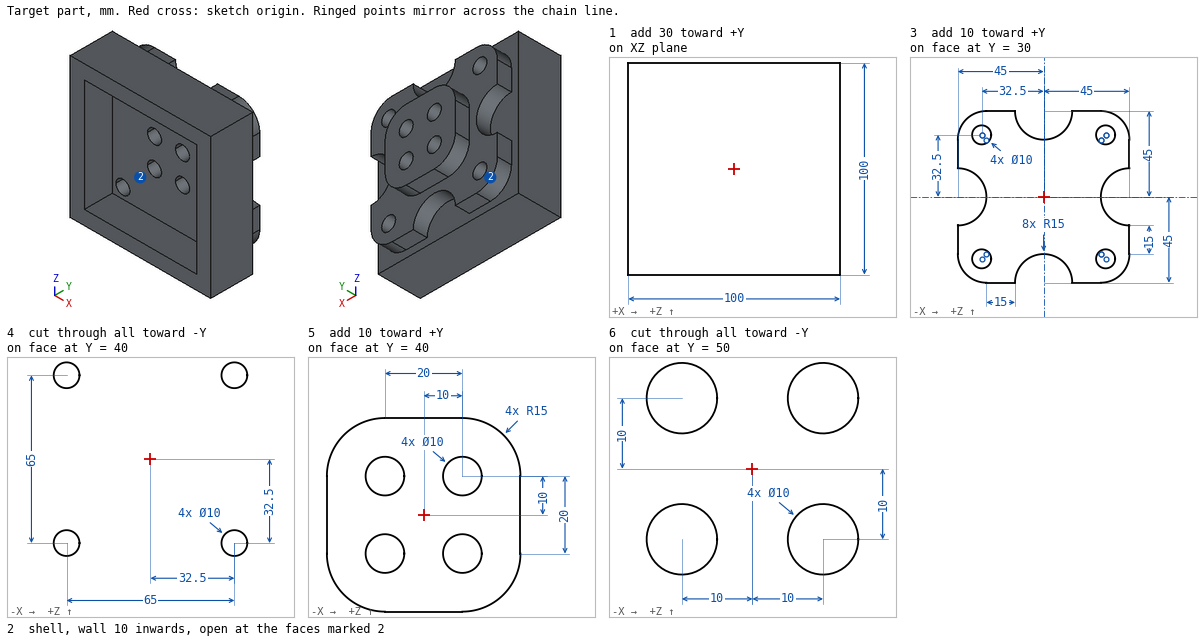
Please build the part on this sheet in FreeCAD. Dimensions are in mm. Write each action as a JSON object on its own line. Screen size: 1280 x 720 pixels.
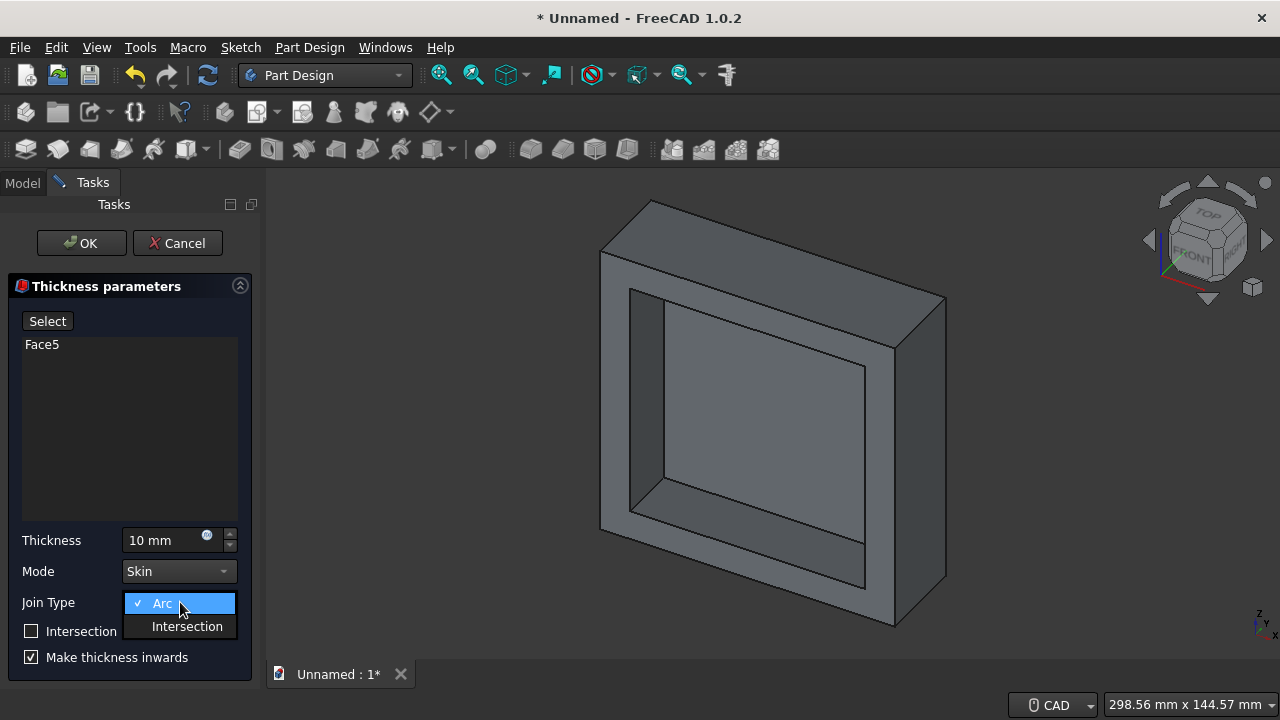
{"action": "left_click", "coordinate": [179, 626]}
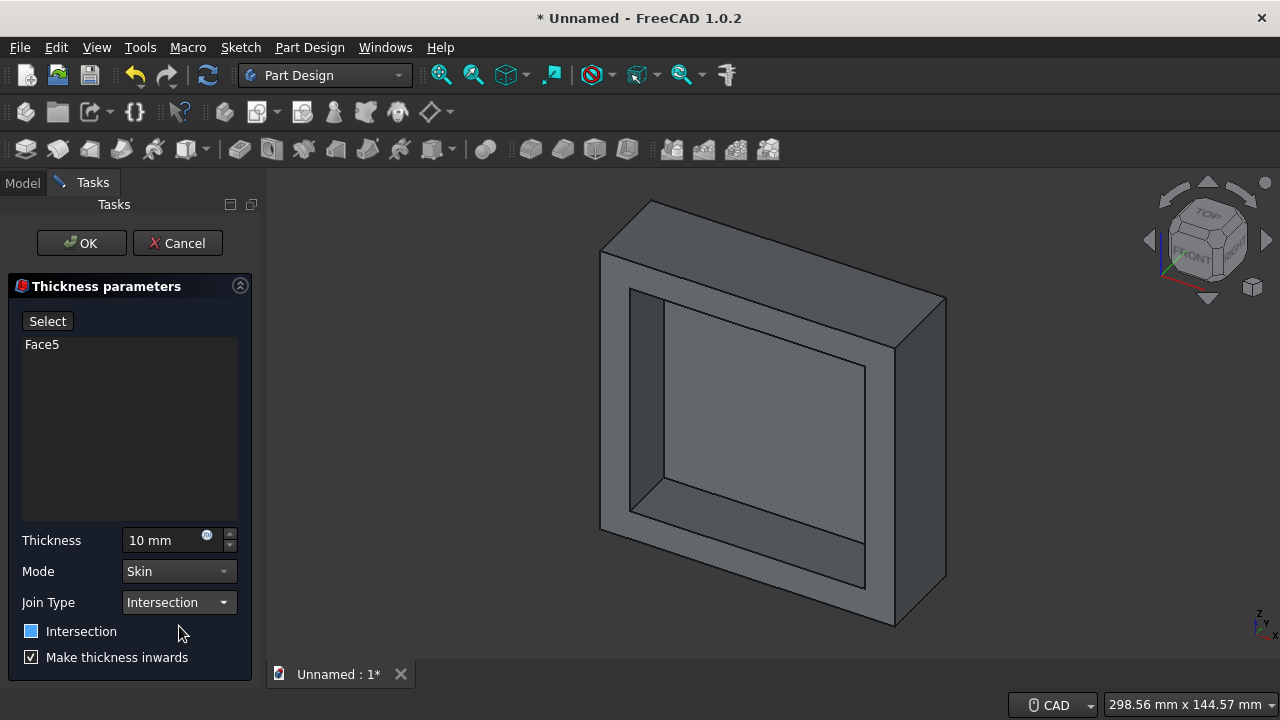
{"action": "left_click", "coordinate": [82, 243]}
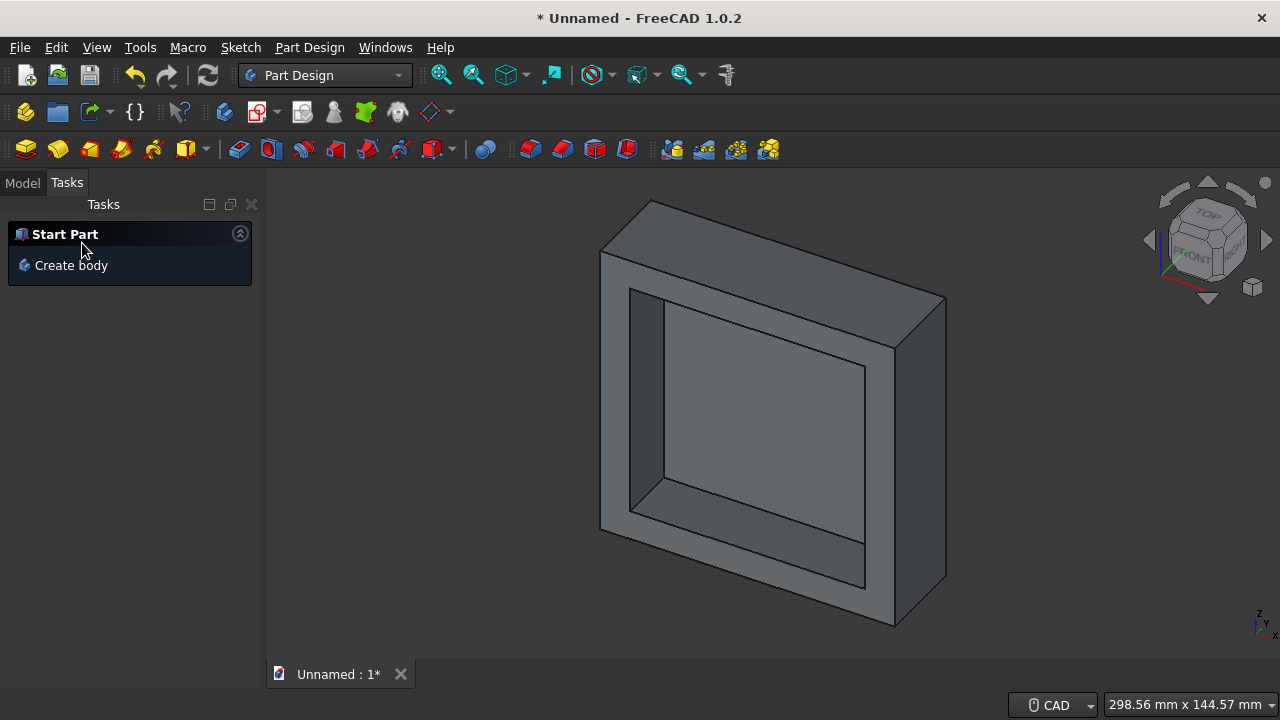
{"action": "key", "text": "4"}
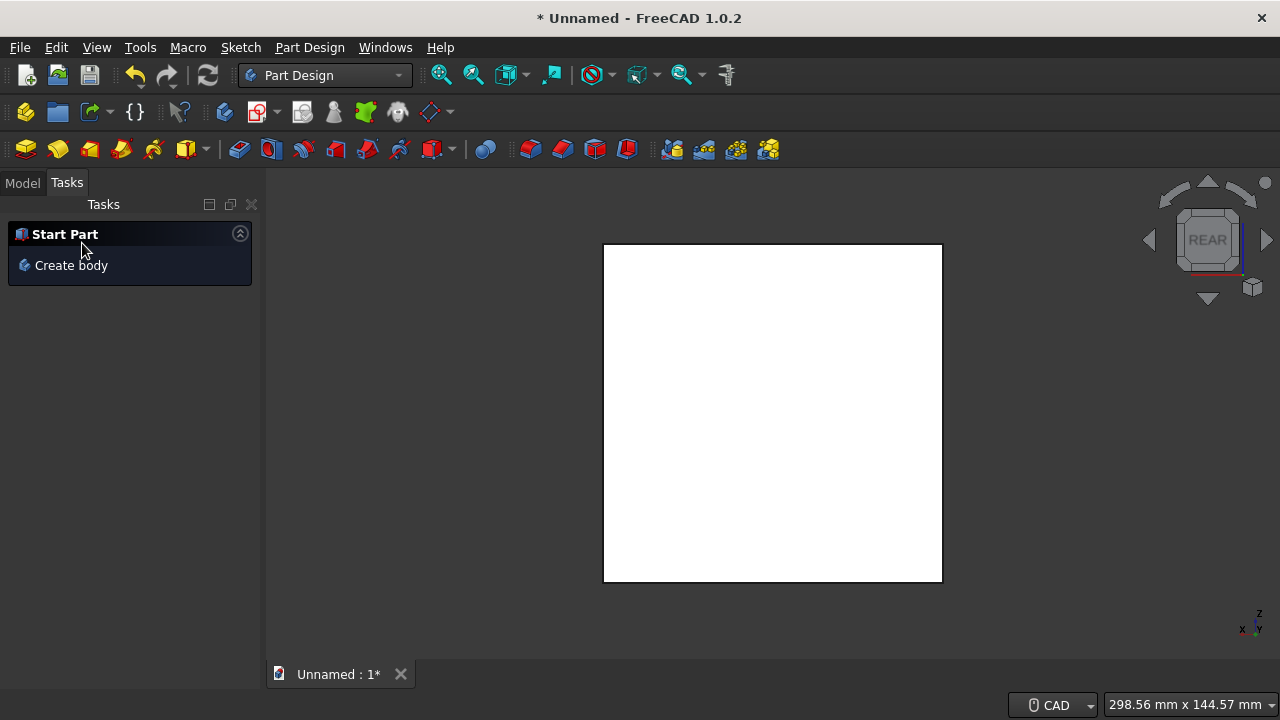
{"action": "left_click", "coordinate": [773, 412]}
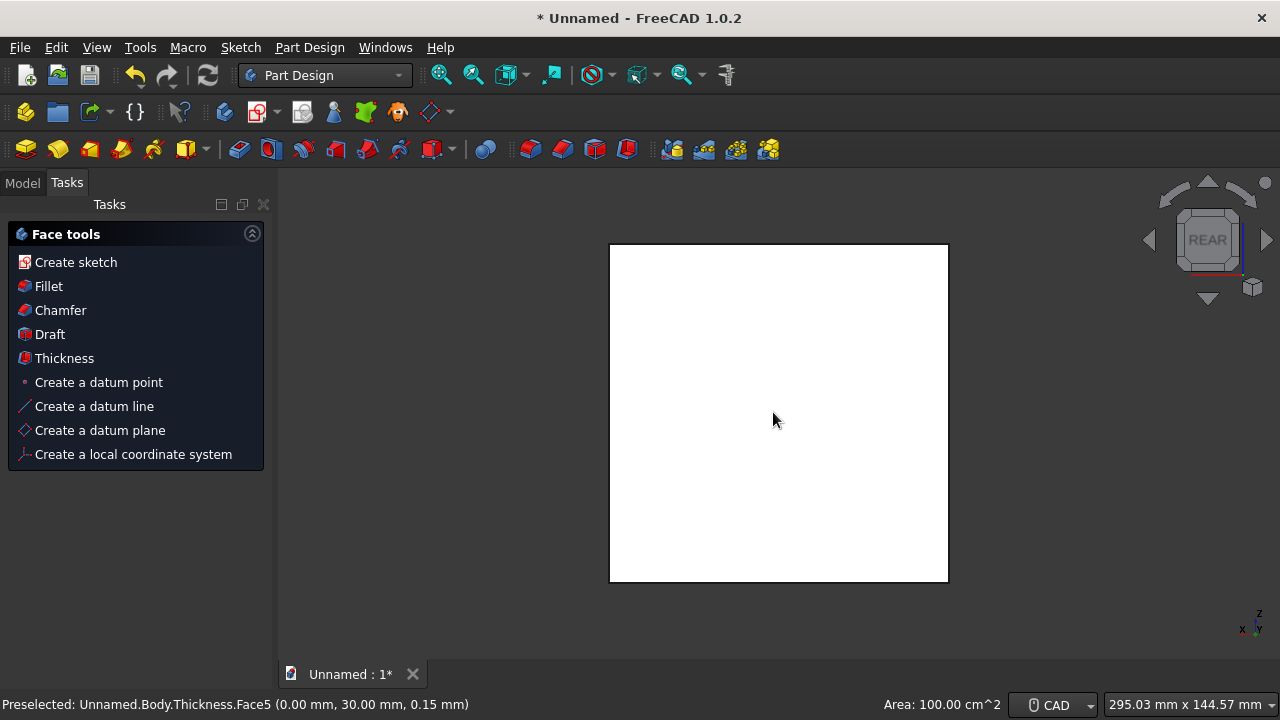
{"action": "left_click", "coordinate": [258, 112]}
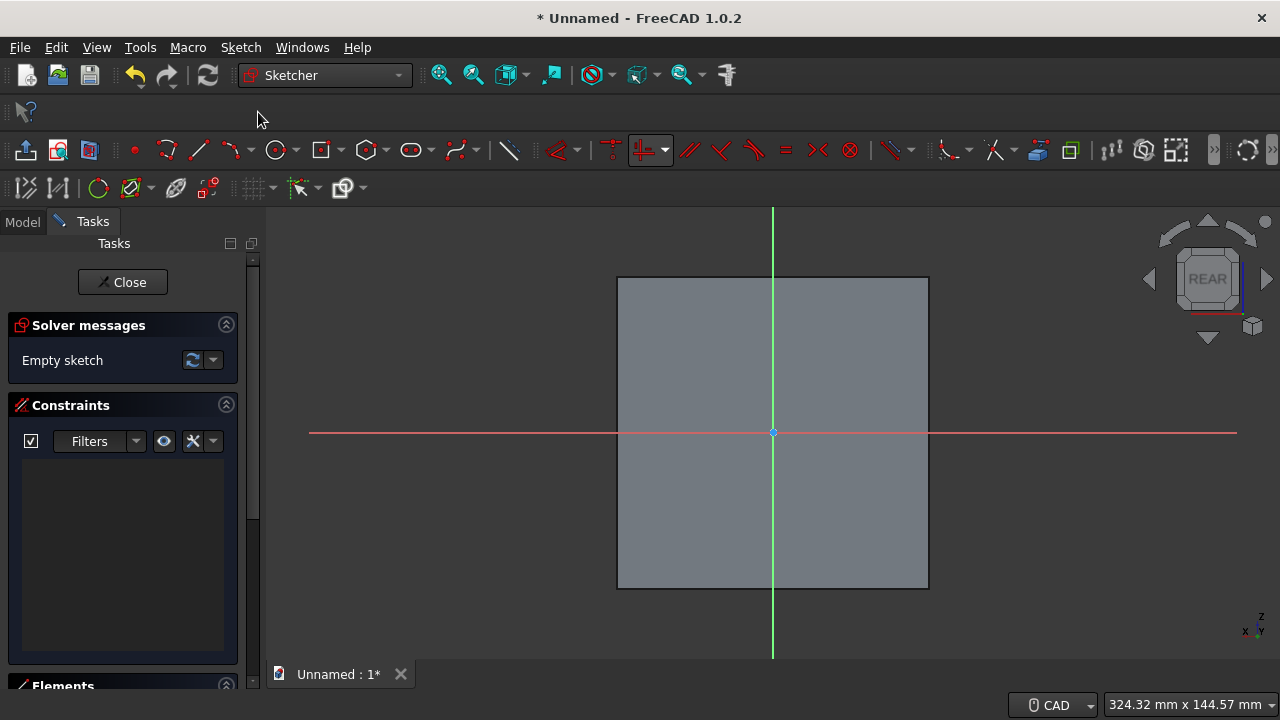
{"action": "left_click", "coordinate": [200, 150]}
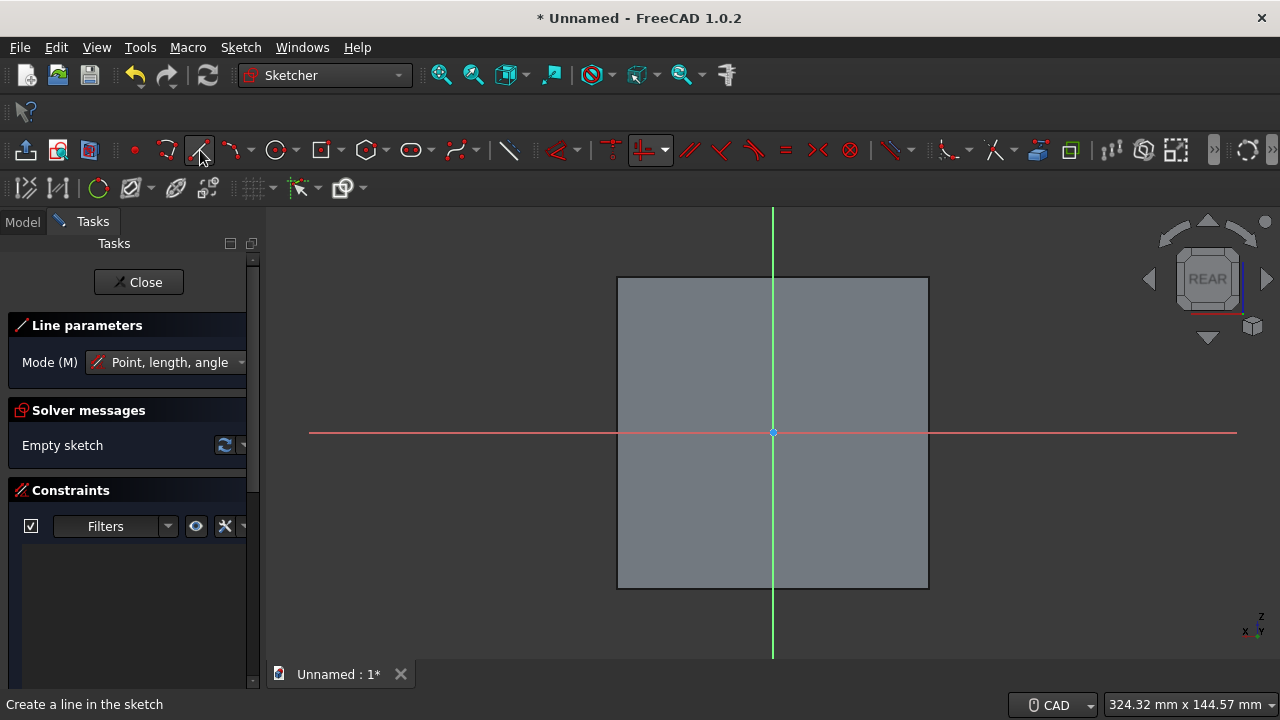
{"action": "left_click", "coordinate": [679, 574]}
{"action": "left_click", "coordinate": [726, 574]}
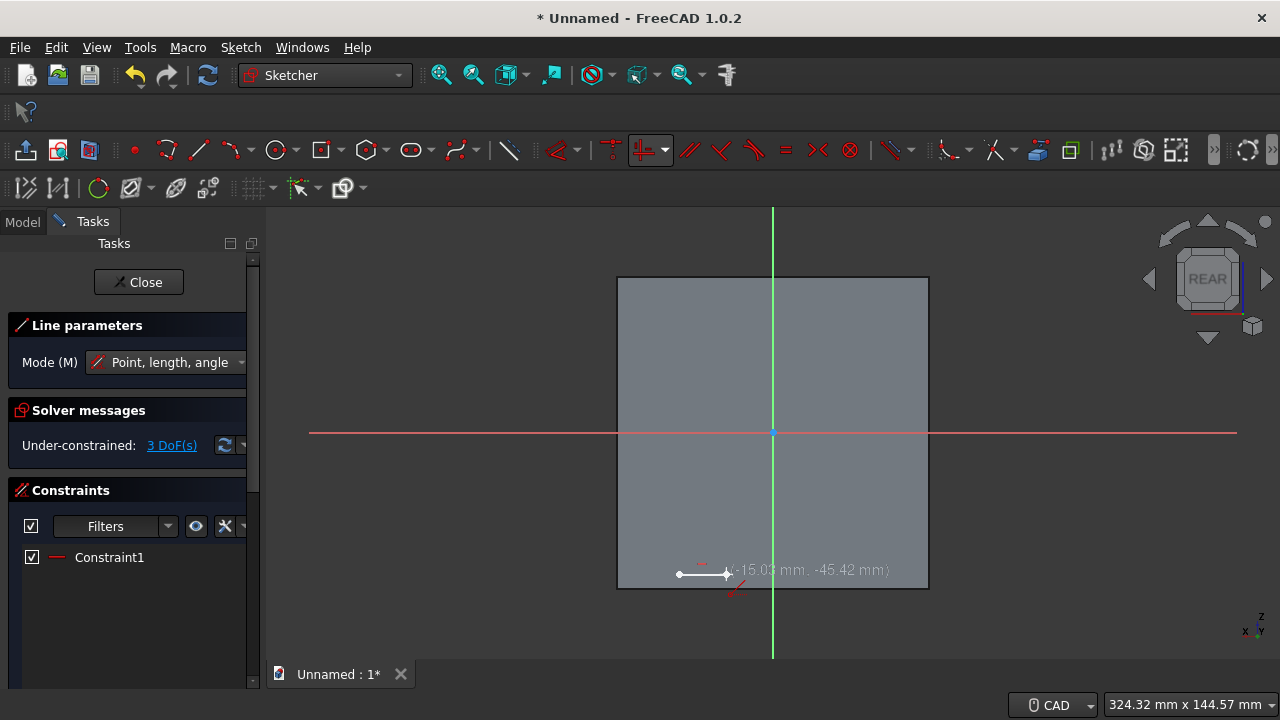
{"action": "left_click", "coordinate": [820, 574]}
{"action": "left_click", "coordinate": [867, 574]}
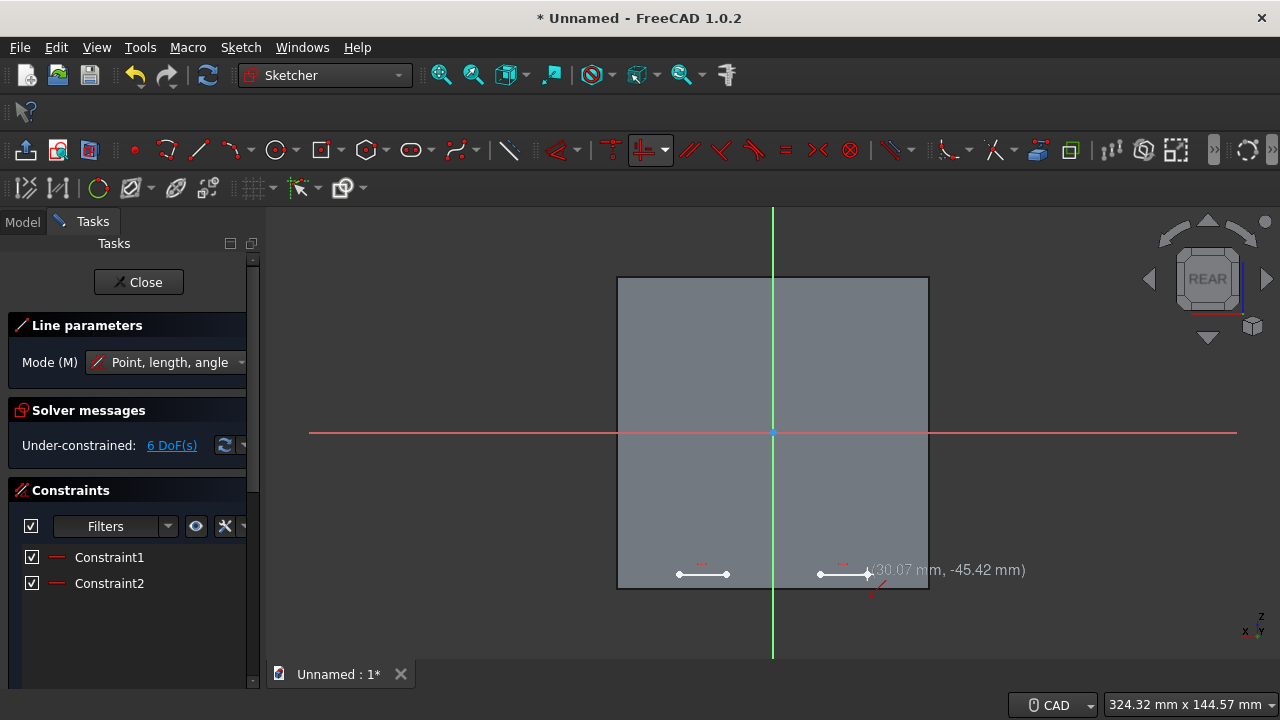
{"action": "left_click", "coordinate": [914, 527]}
{"action": "left_click", "coordinate": [914, 480]}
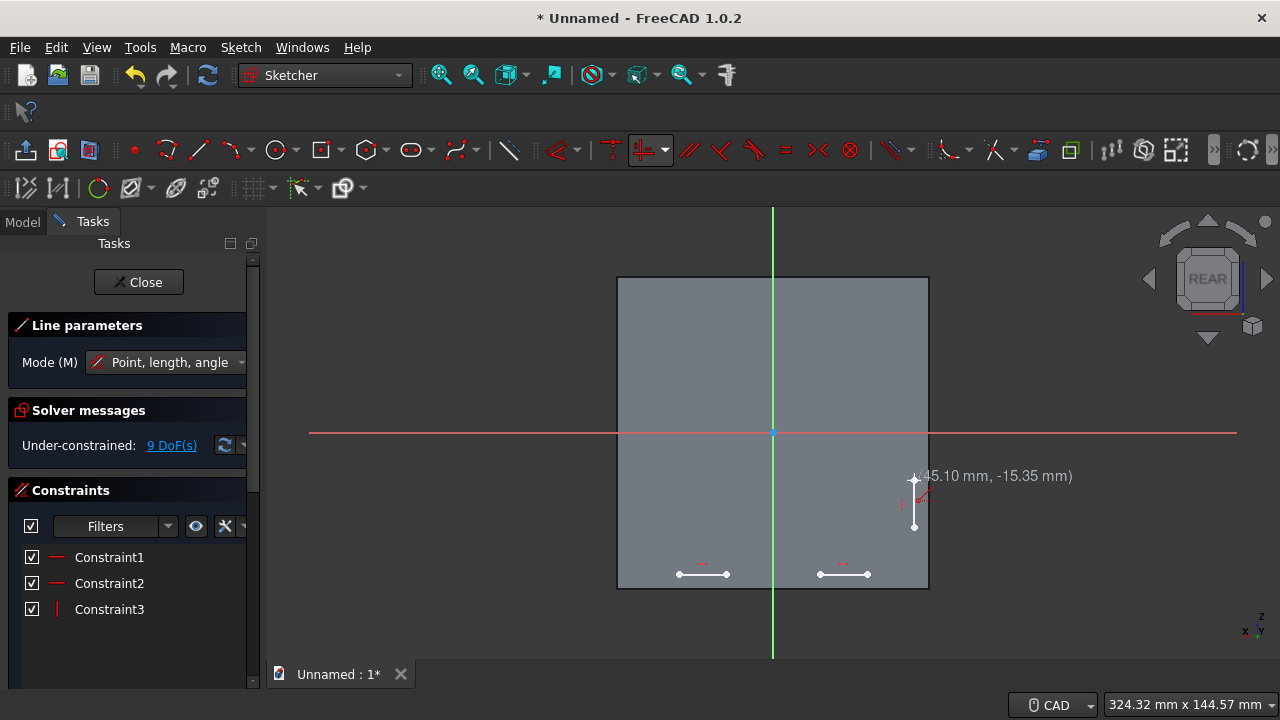
{"action": "left_click", "coordinate": [914, 386]}
{"action": "left_click", "coordinate": [914, 339]}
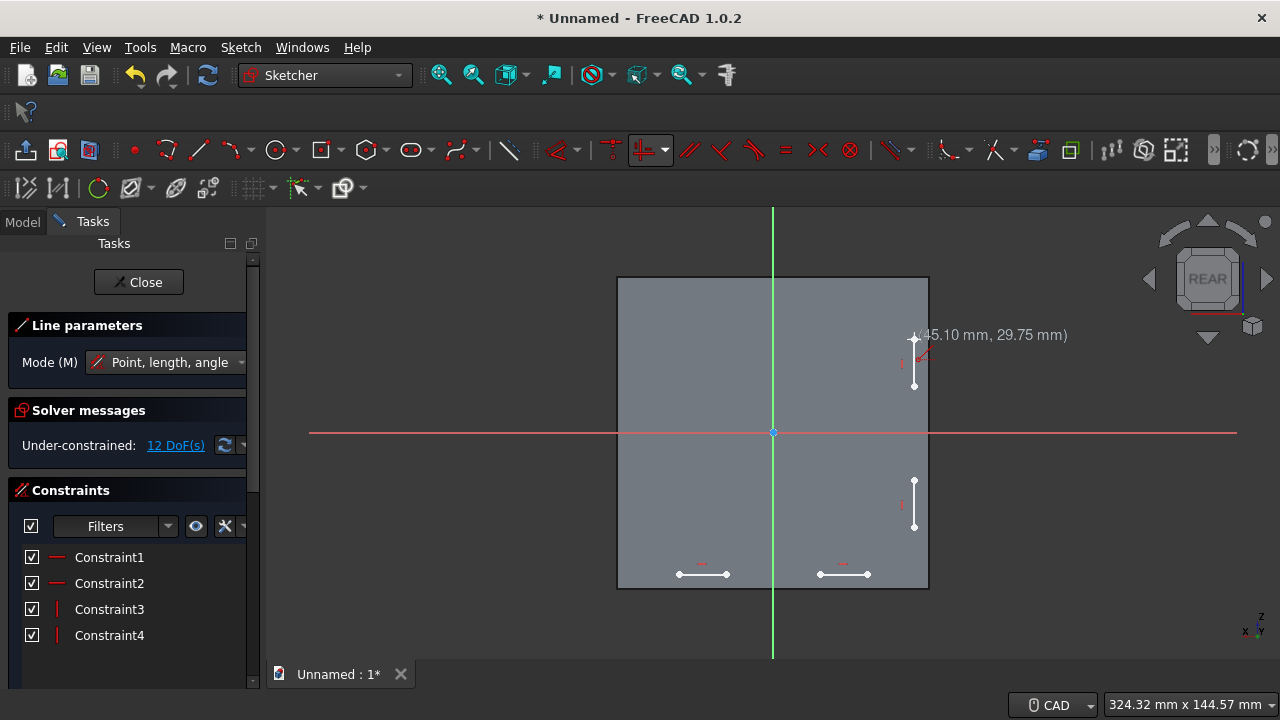
{"action": "left_click", "coordinate": [867, 292]}
{"action": "left_click", "coordinate": [820, 292]}